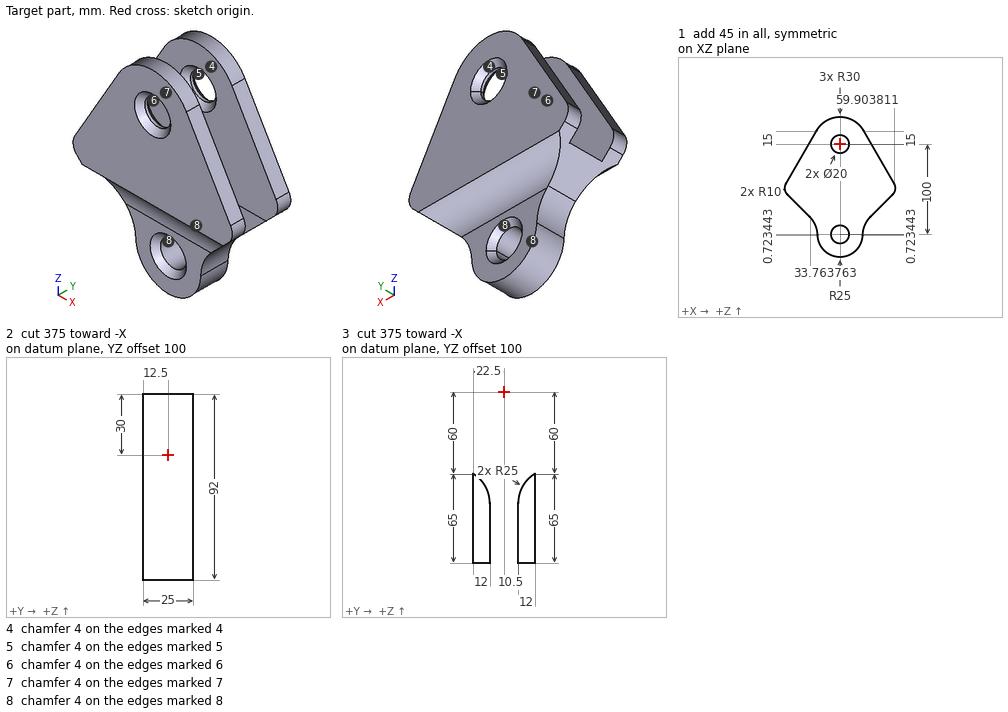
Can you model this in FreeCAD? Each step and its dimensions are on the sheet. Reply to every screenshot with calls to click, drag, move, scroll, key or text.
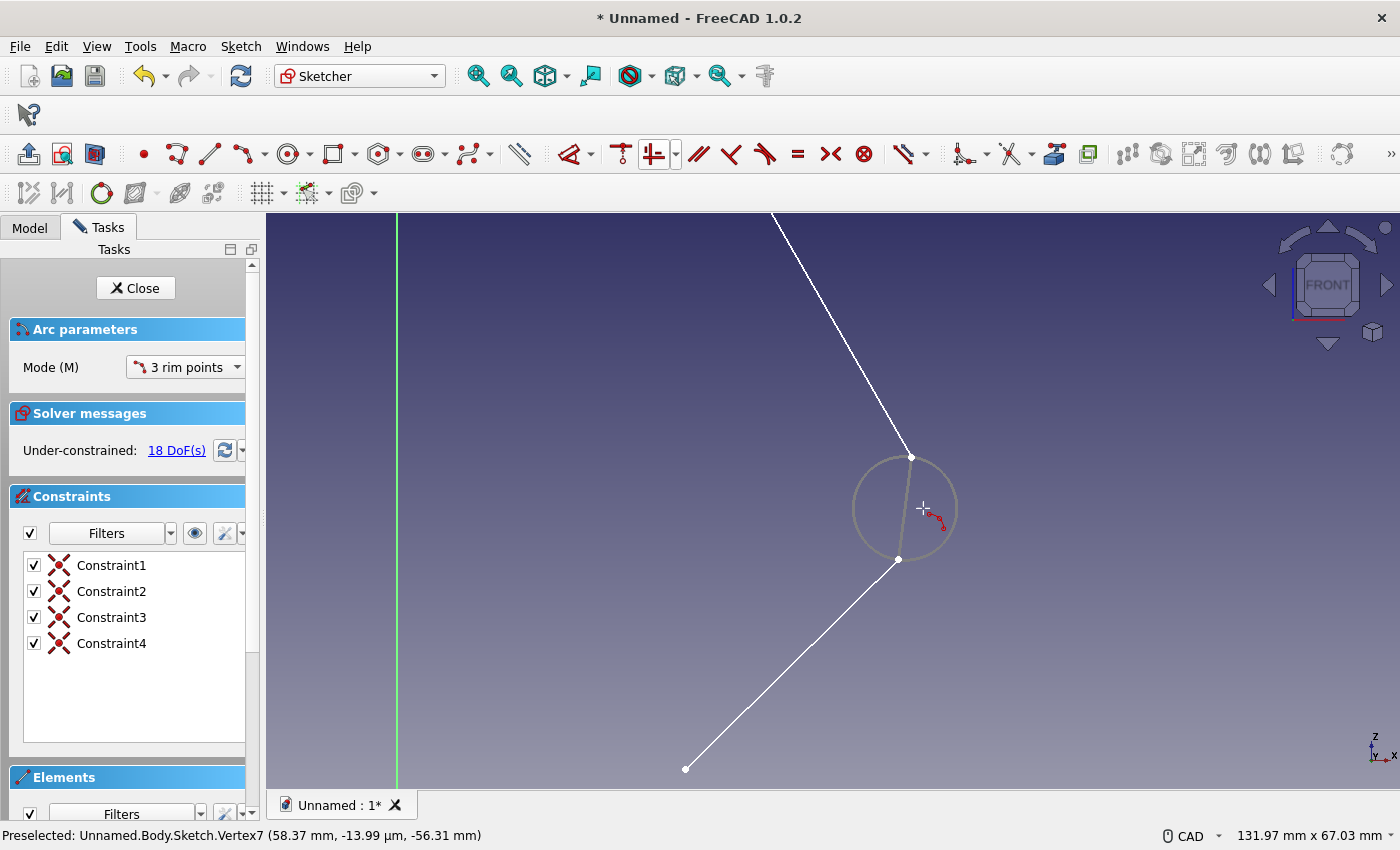
click(922, 506)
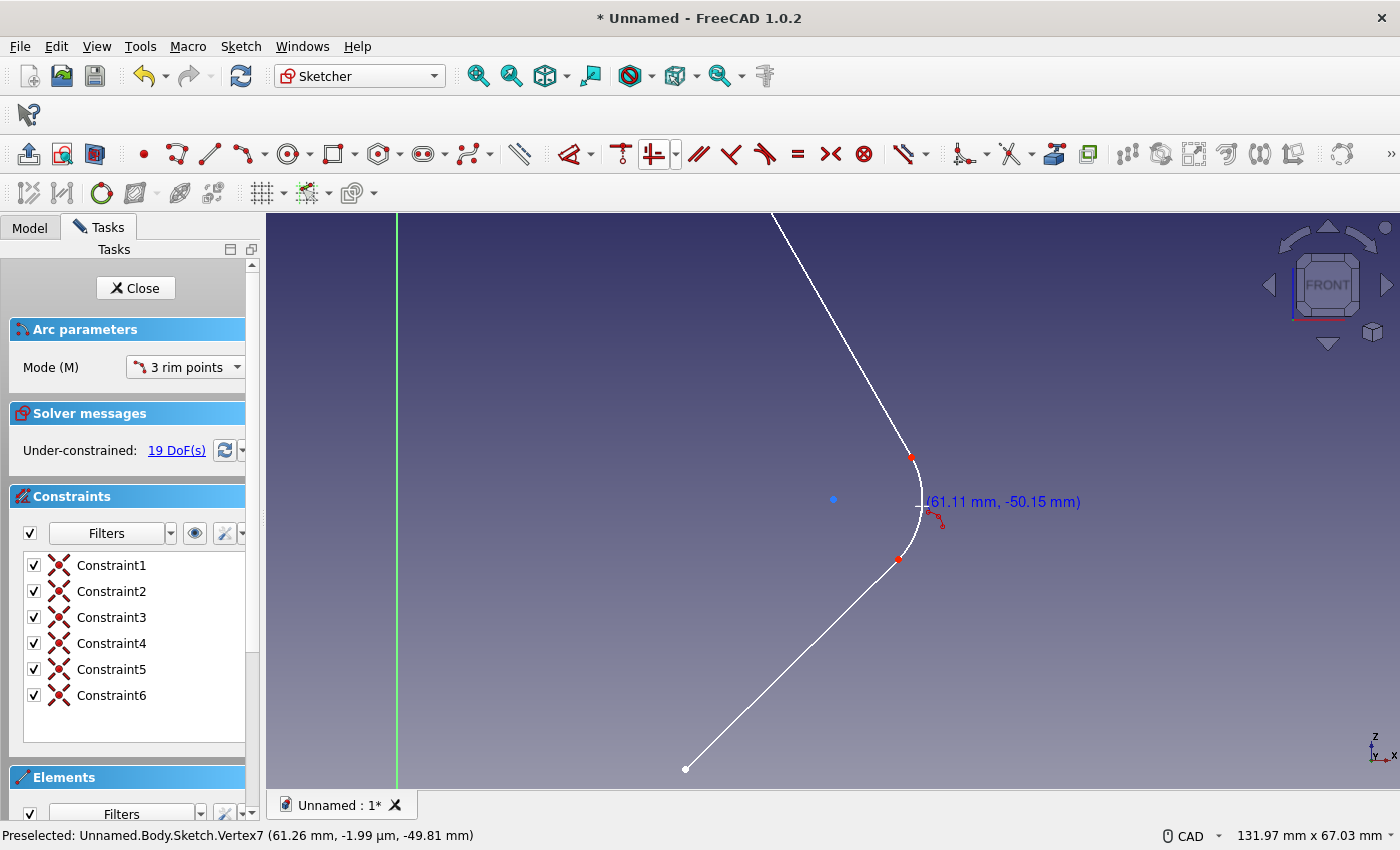
scroll(923, 508, down, 6)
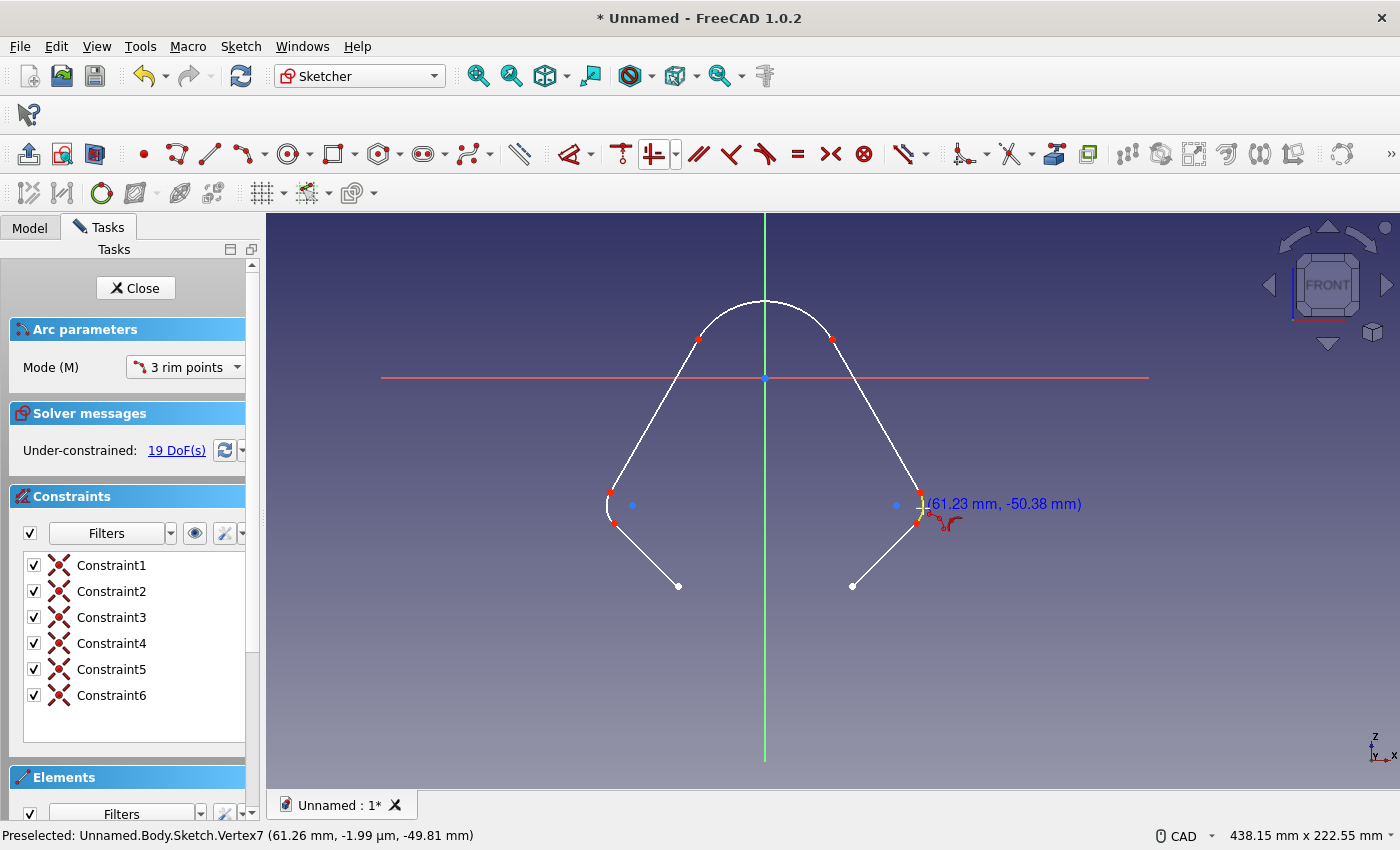
click(852, 587)
click(830, 639)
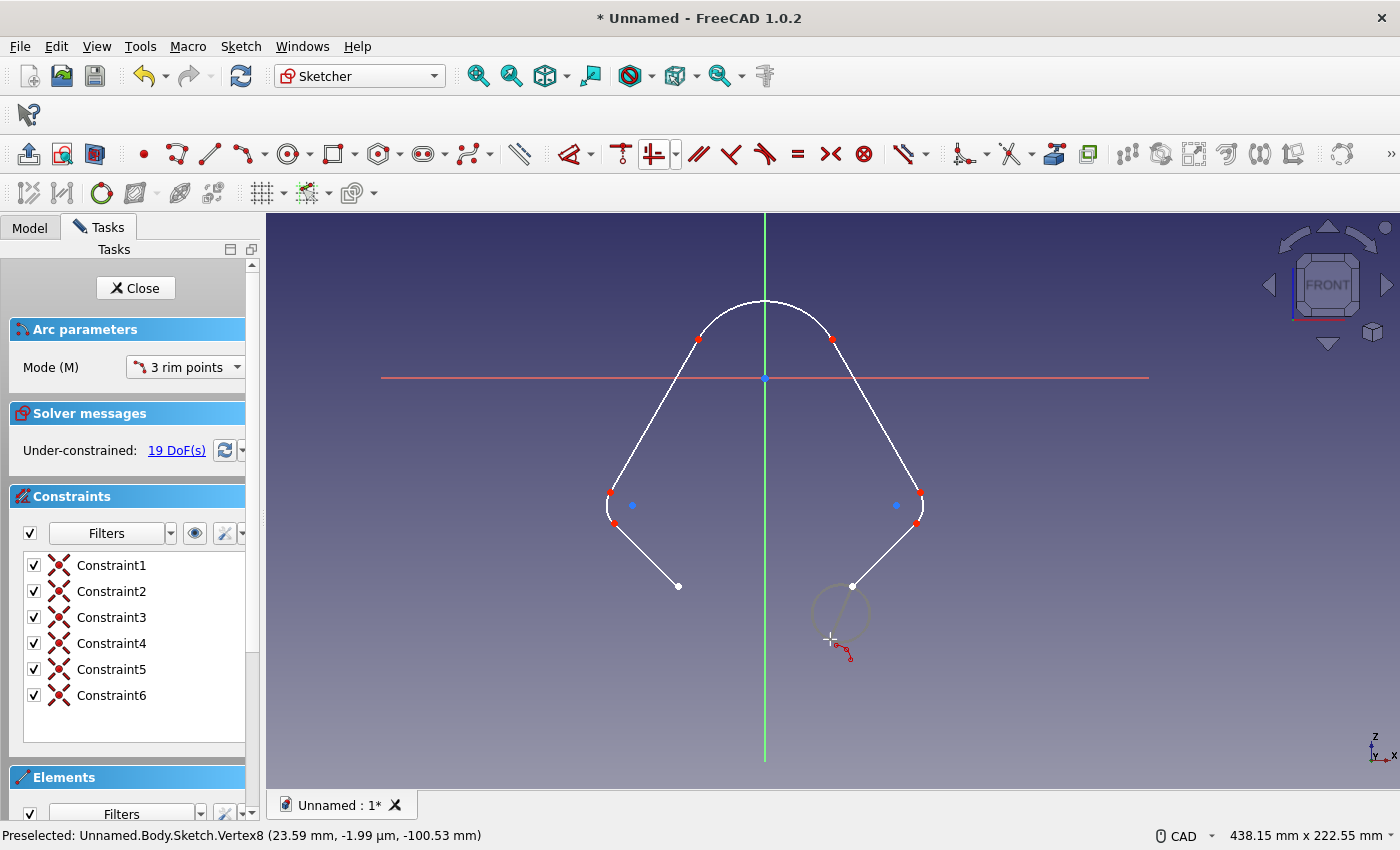
scroll(836, 610, up, 6)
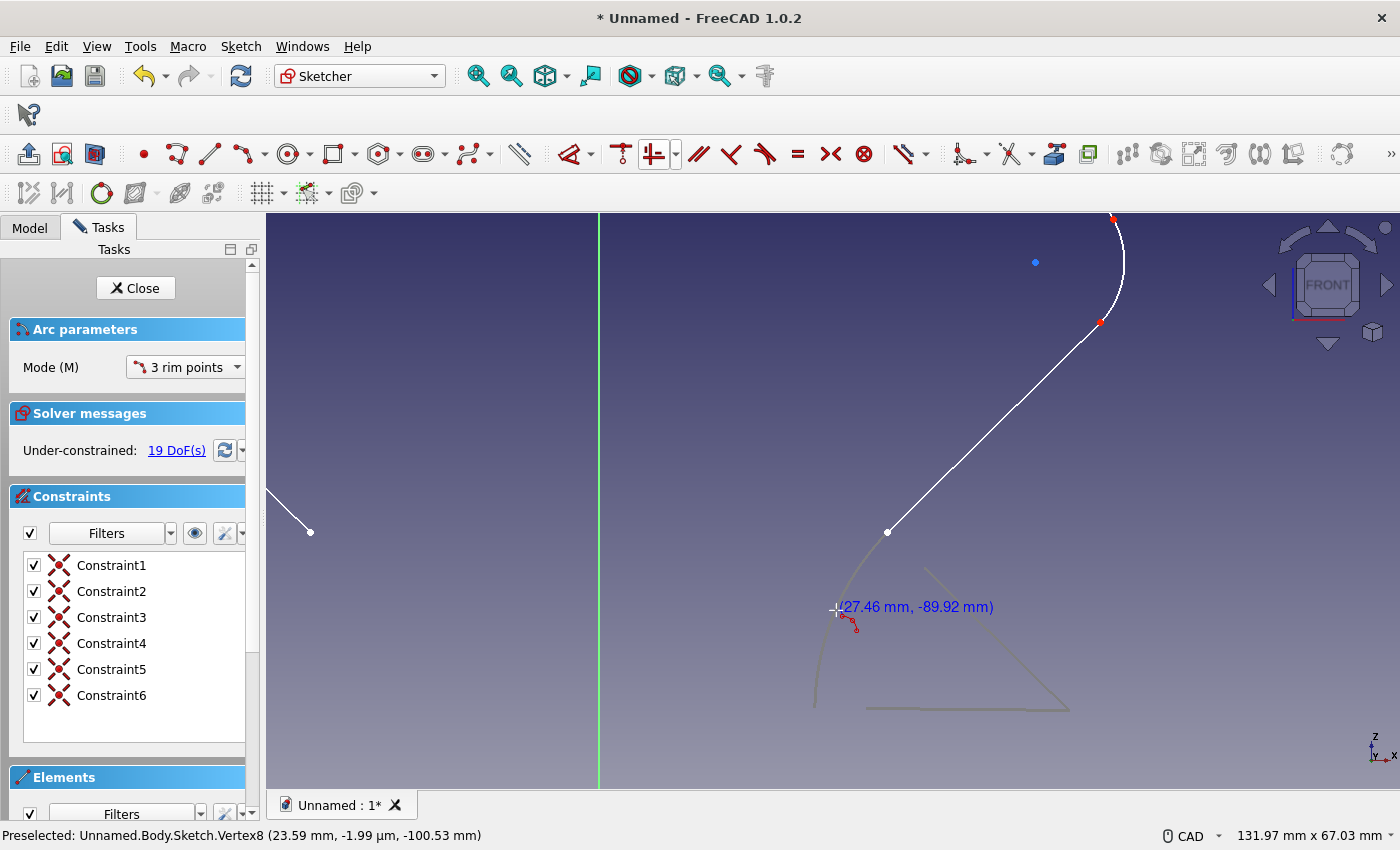
click(835, 610)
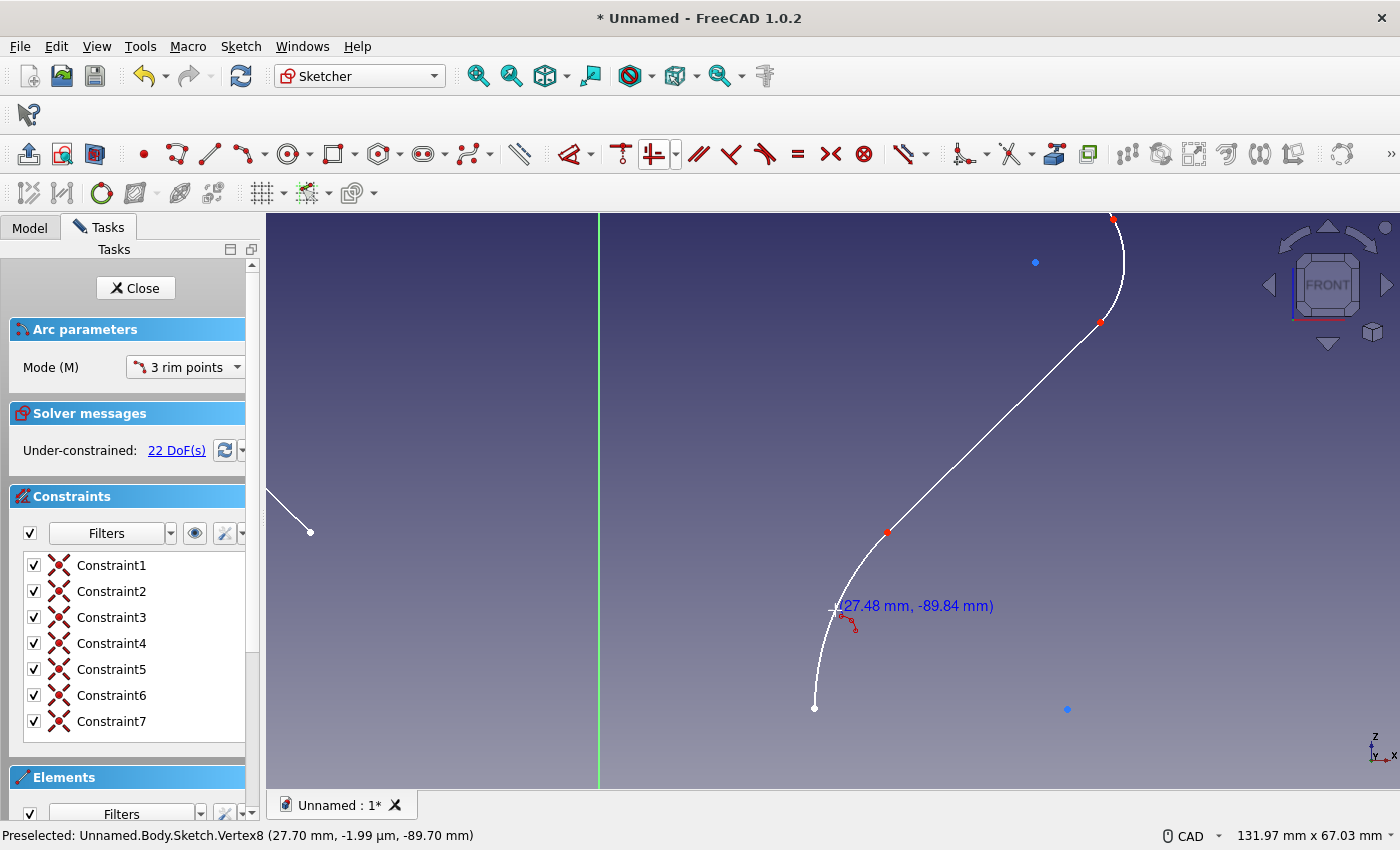
click(815, 708)
click(384, 705)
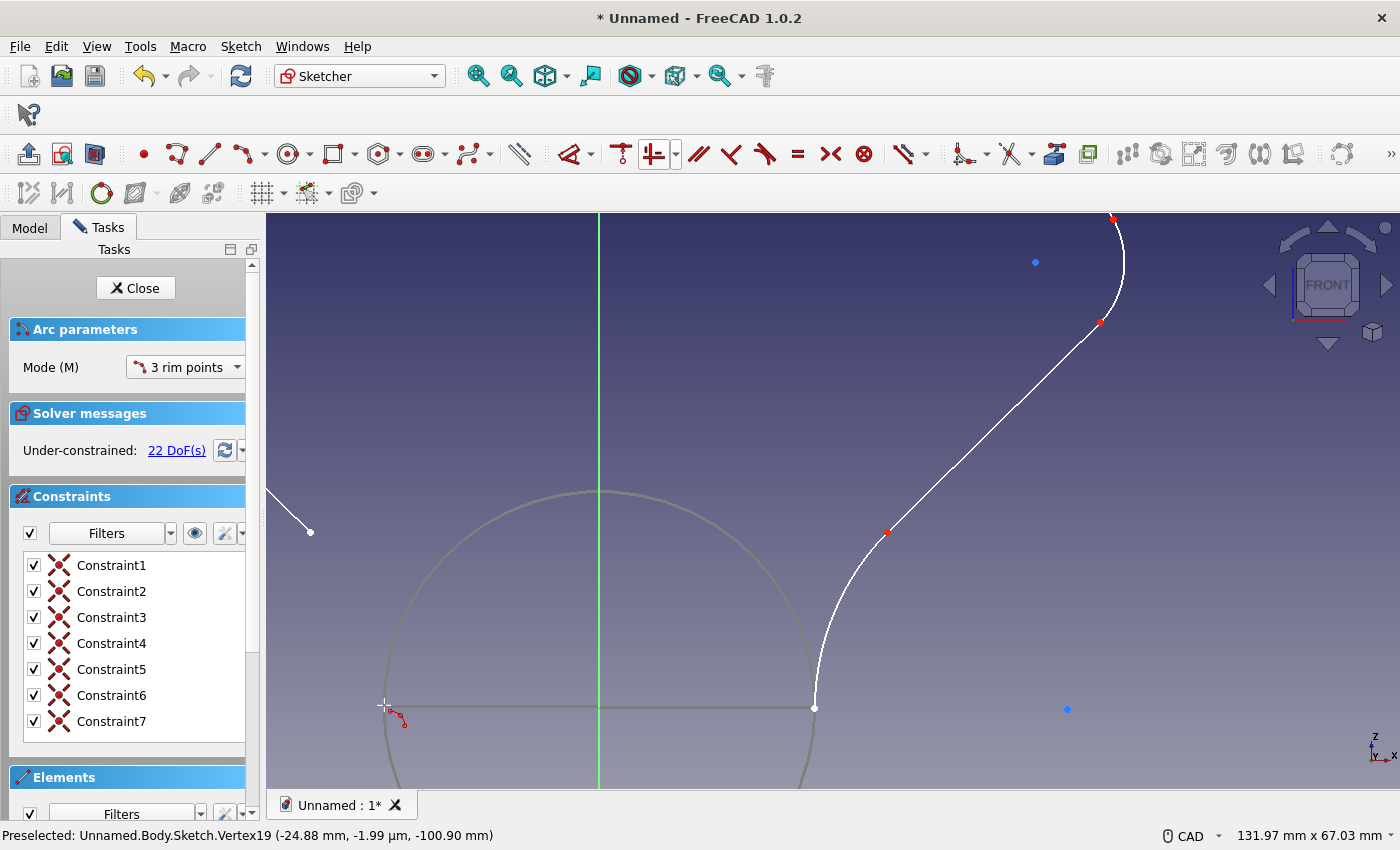
scroll(836, 610, down, 6)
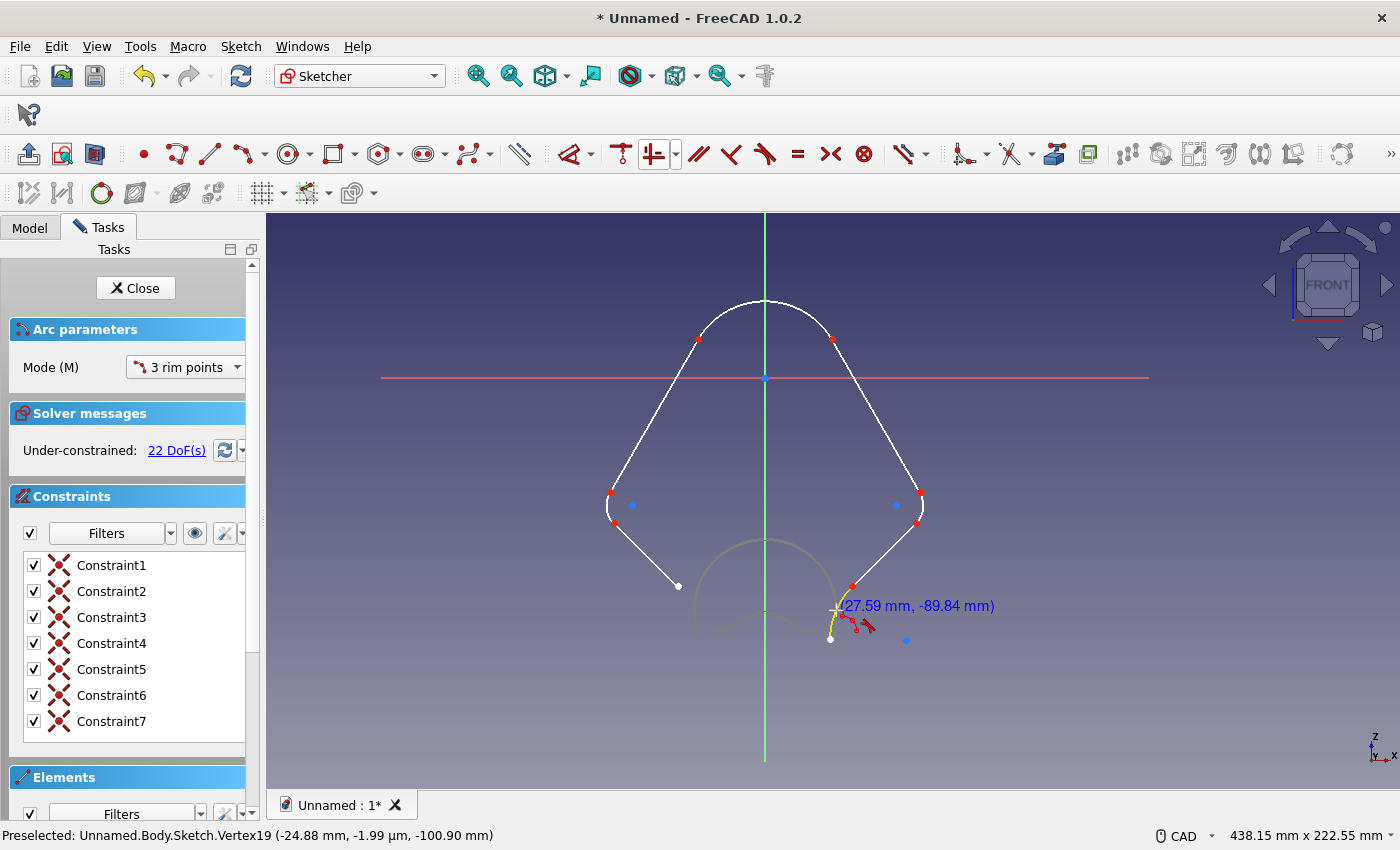
click(745, 699)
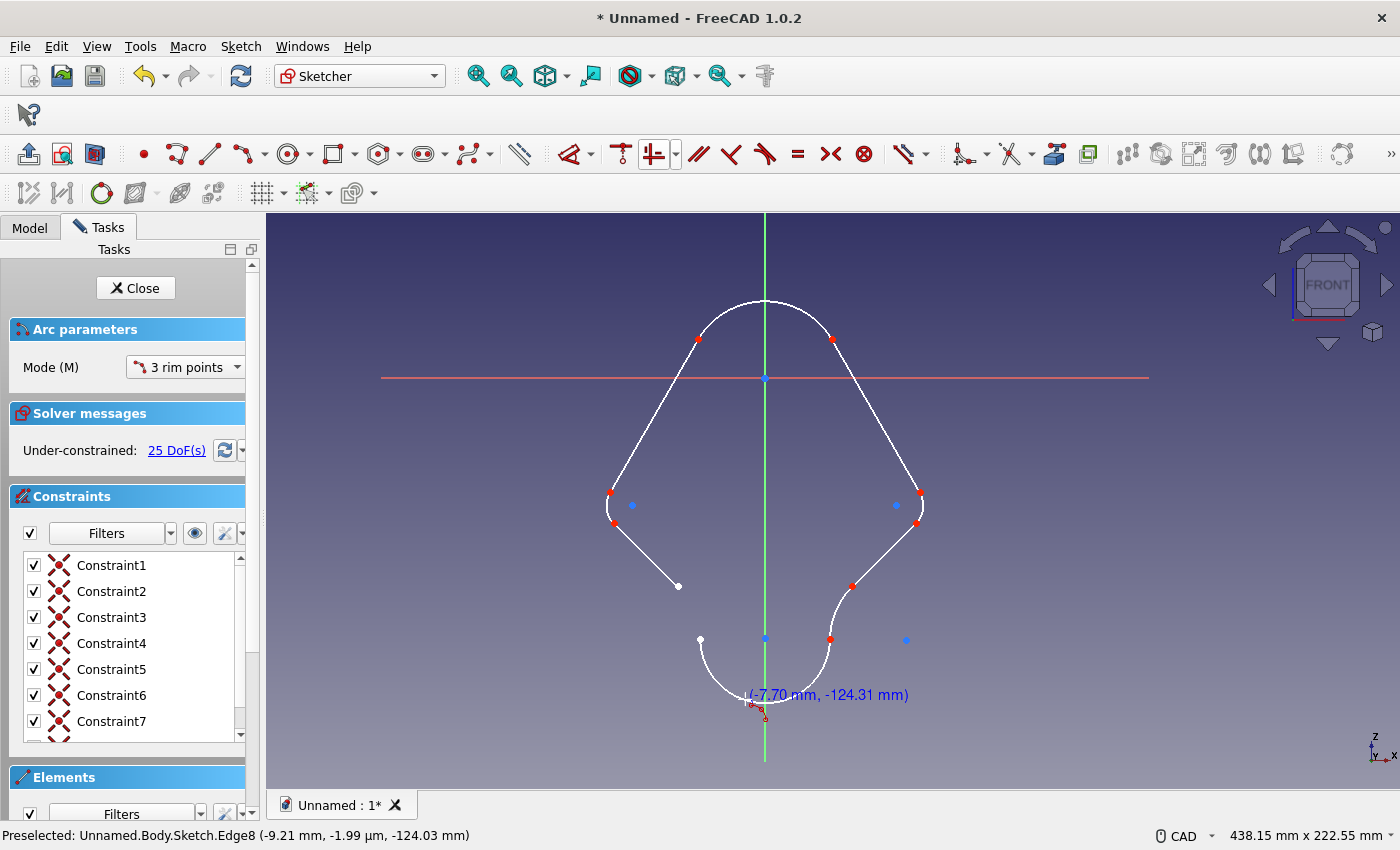
click(700, 639)
click(678, 587)